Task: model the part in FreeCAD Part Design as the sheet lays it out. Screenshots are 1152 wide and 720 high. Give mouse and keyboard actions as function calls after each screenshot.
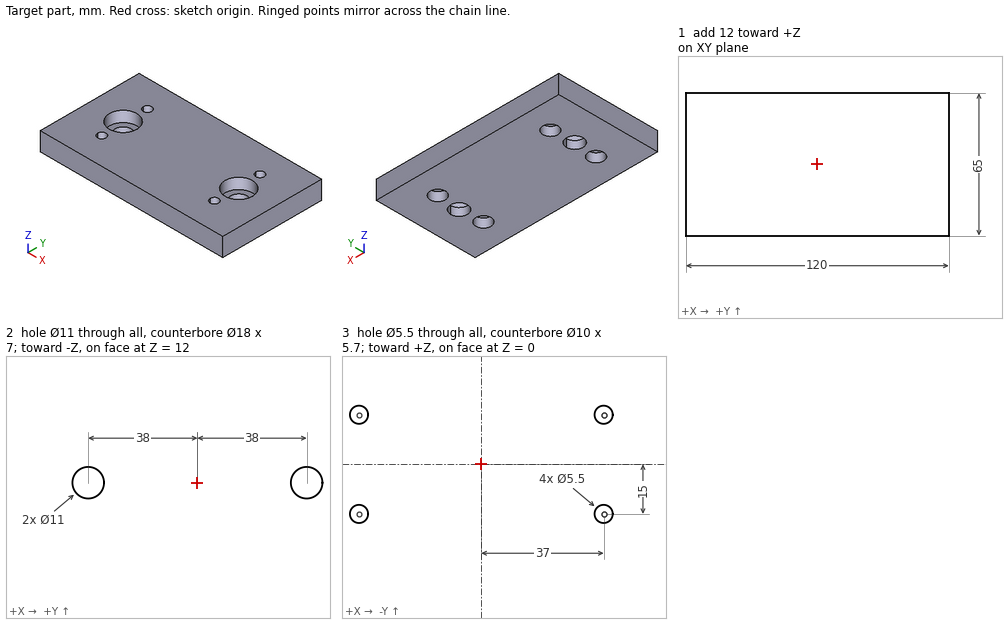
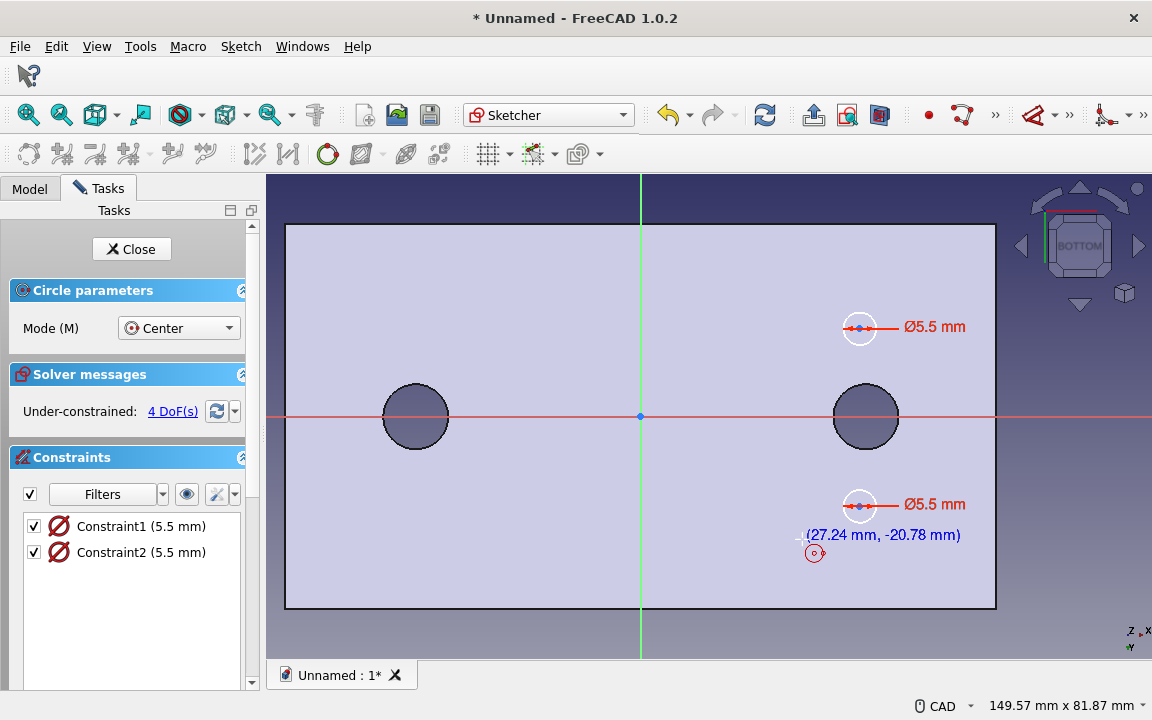
scroll(422, 328, up, 2)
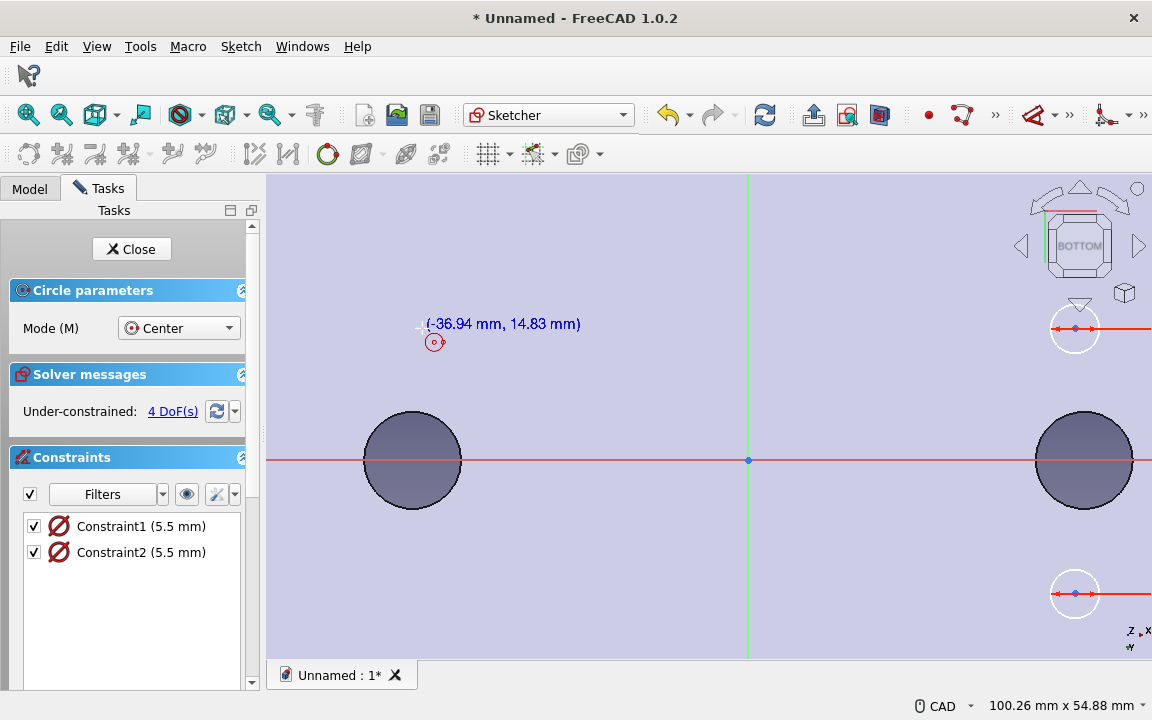
click(421, 328)
move(439, 311)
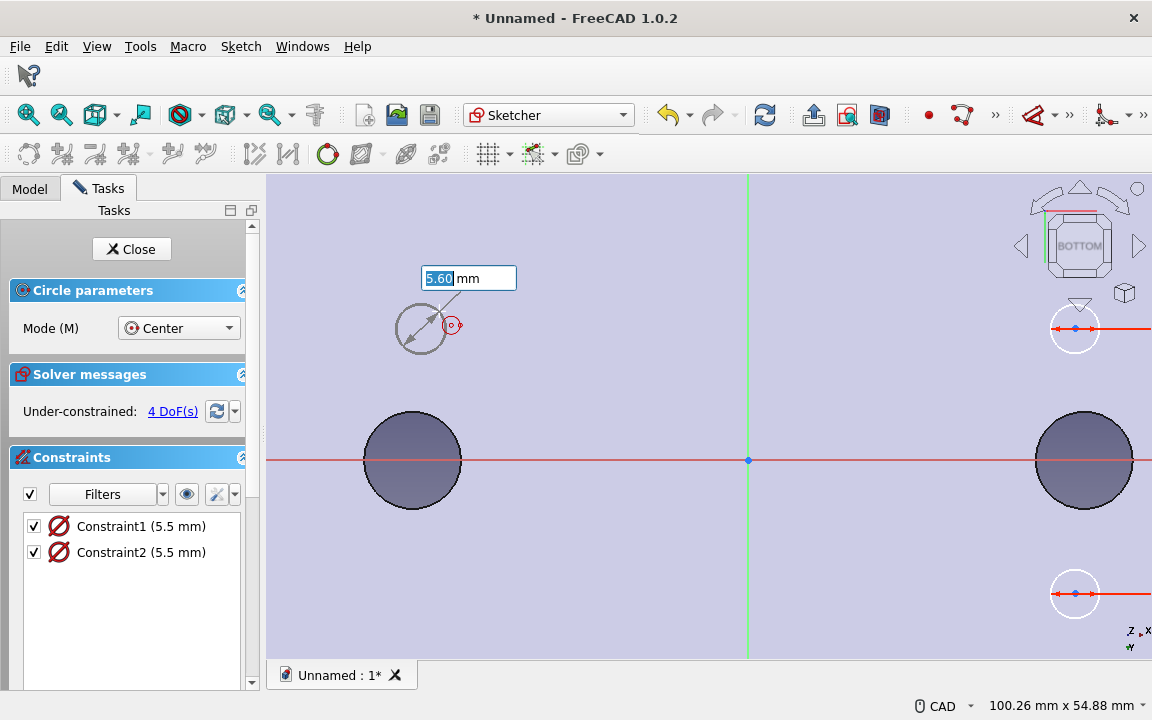
text(5.5)
key(Return)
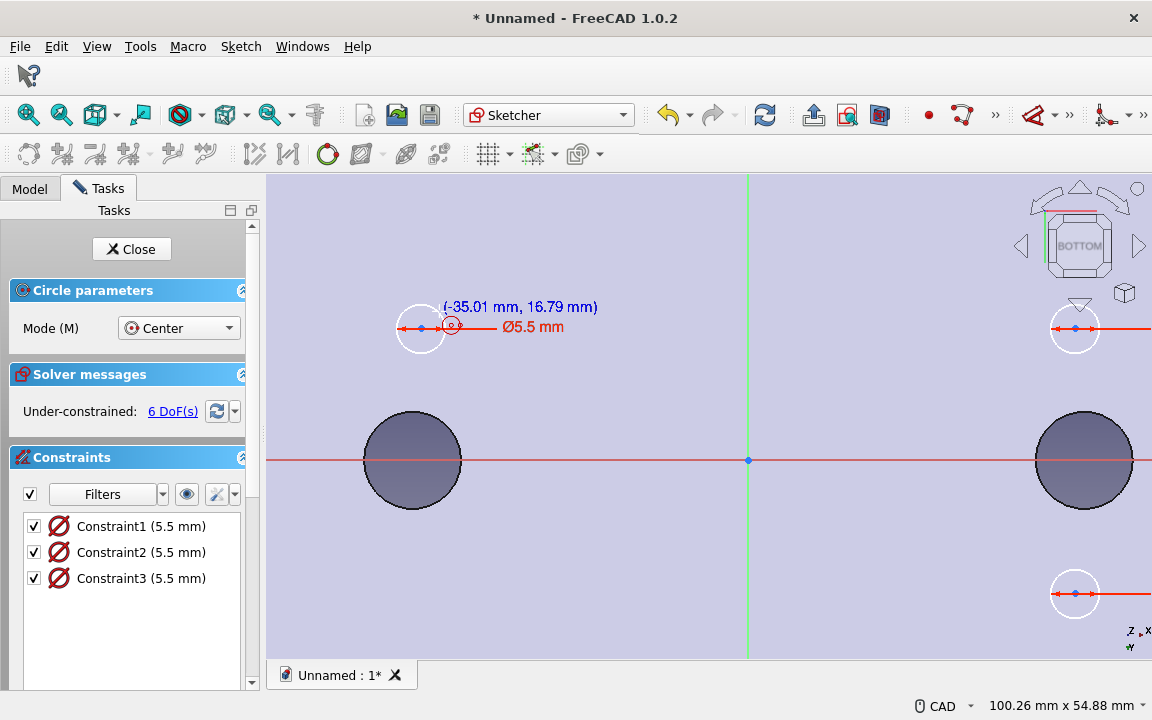
click(421, 593)
move(439, 576)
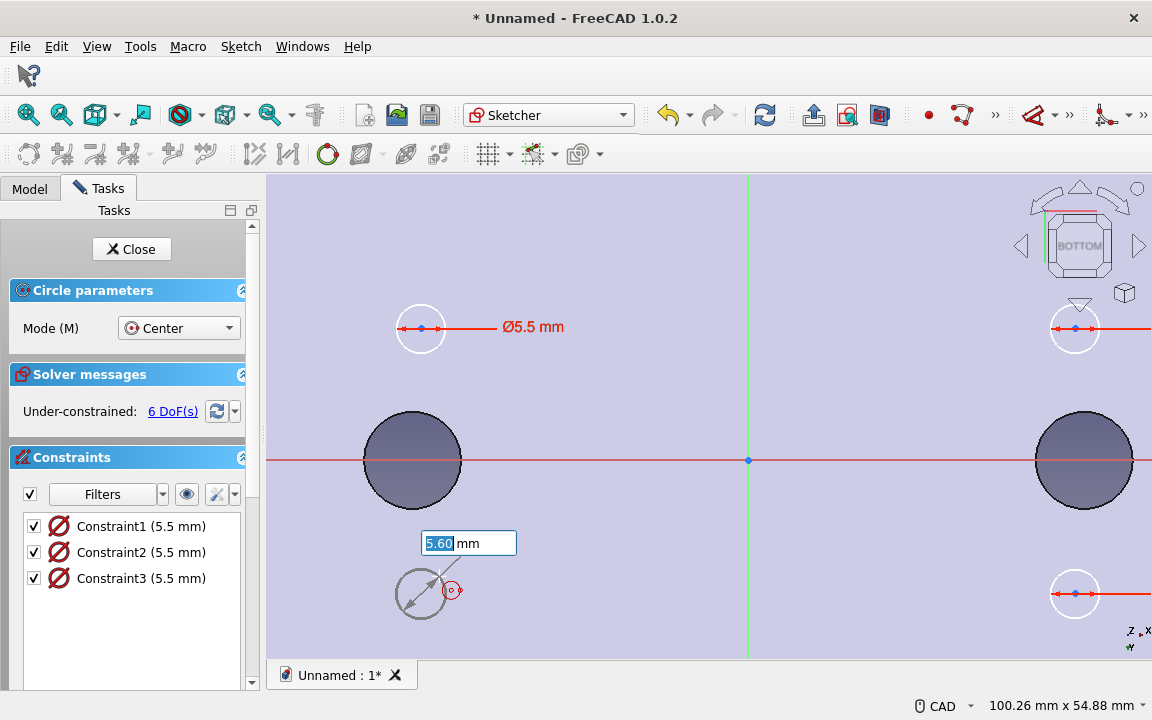
text(5.5)
key(Return)
key(Escape)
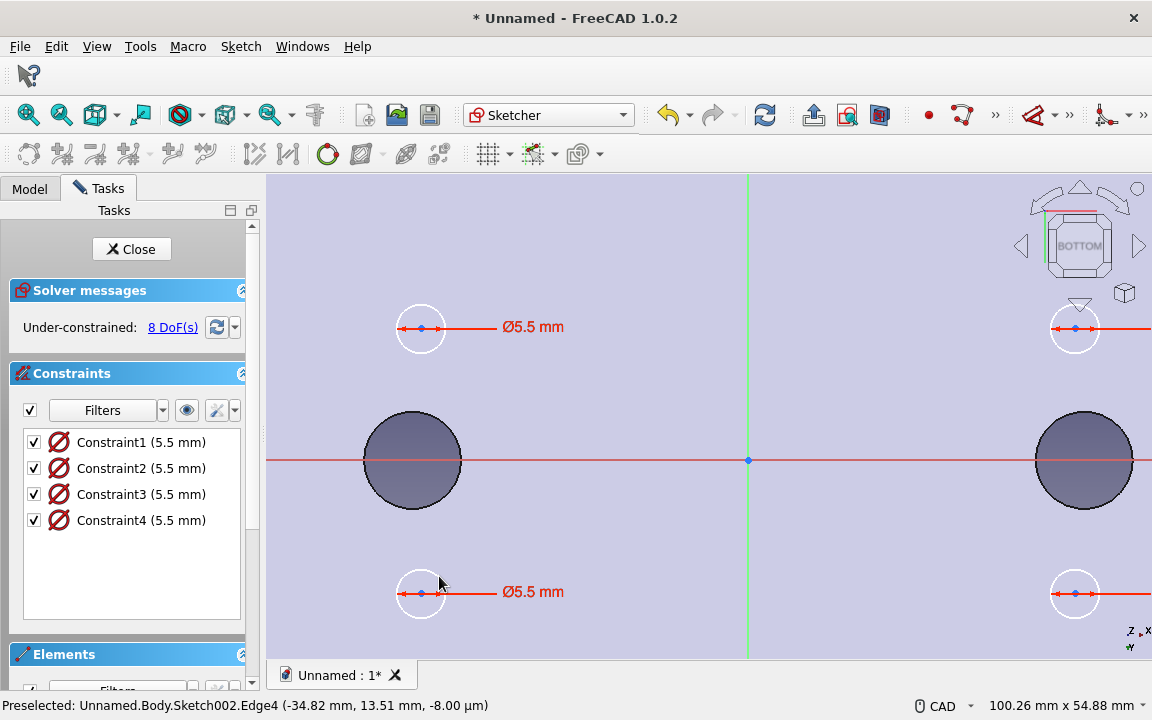
scroll(421, 327, down, 2)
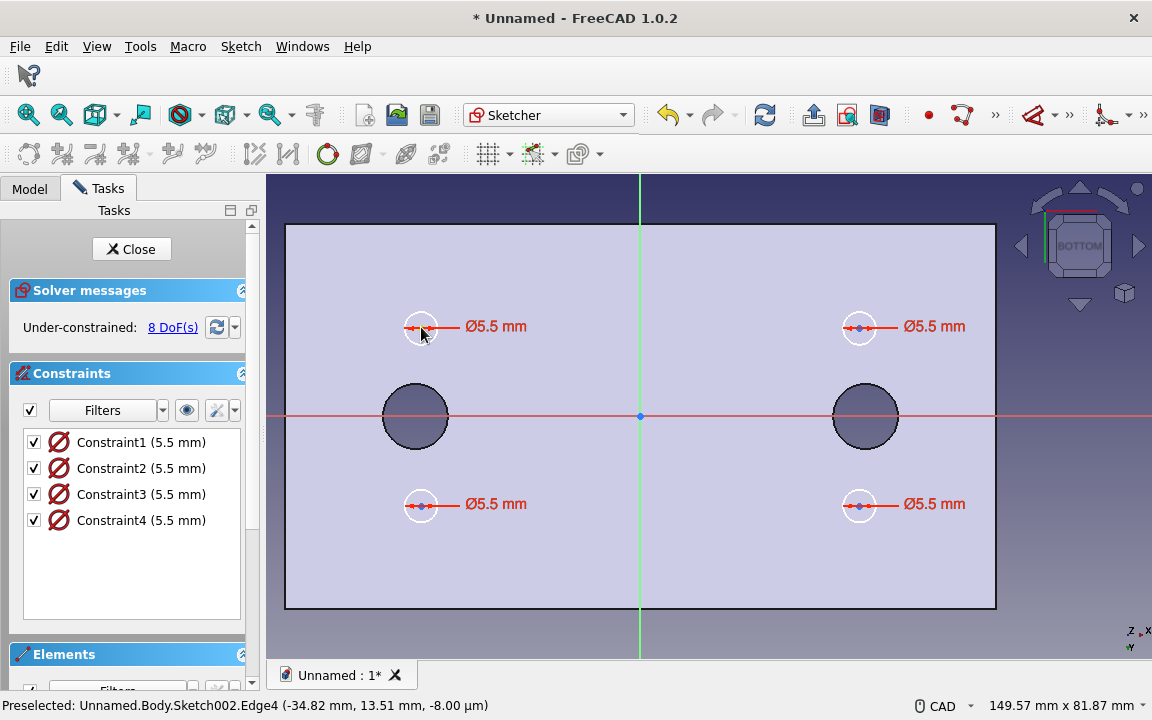
click(860, 506)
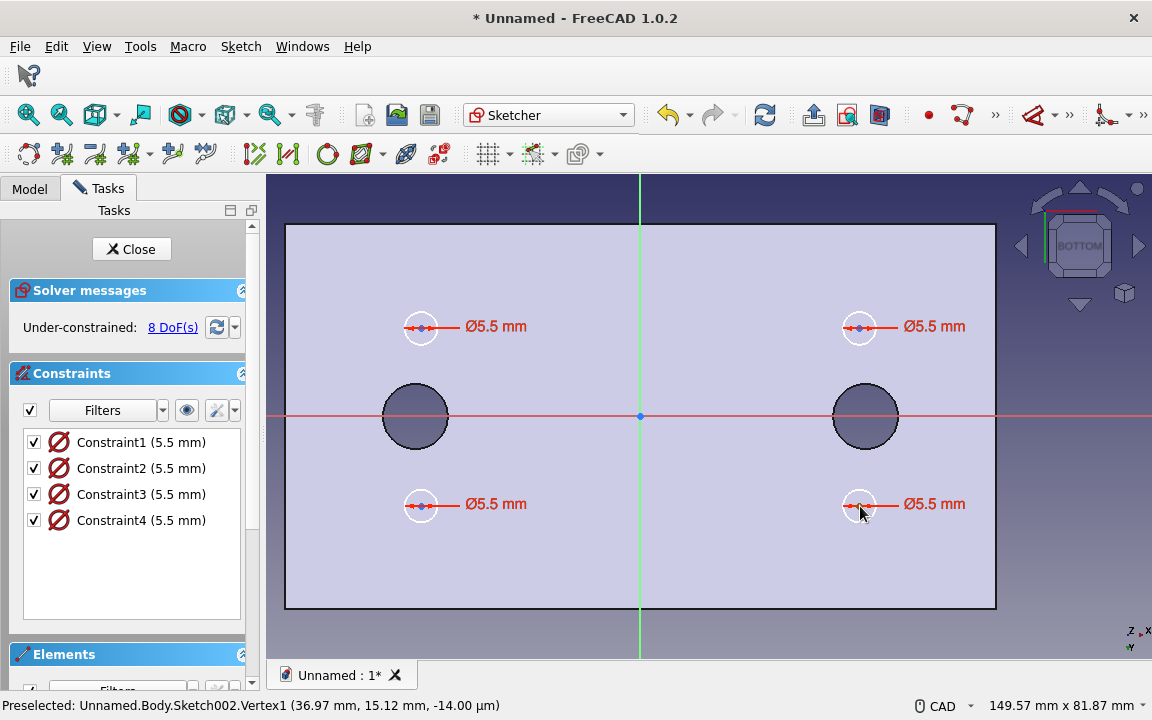
click(860, 328)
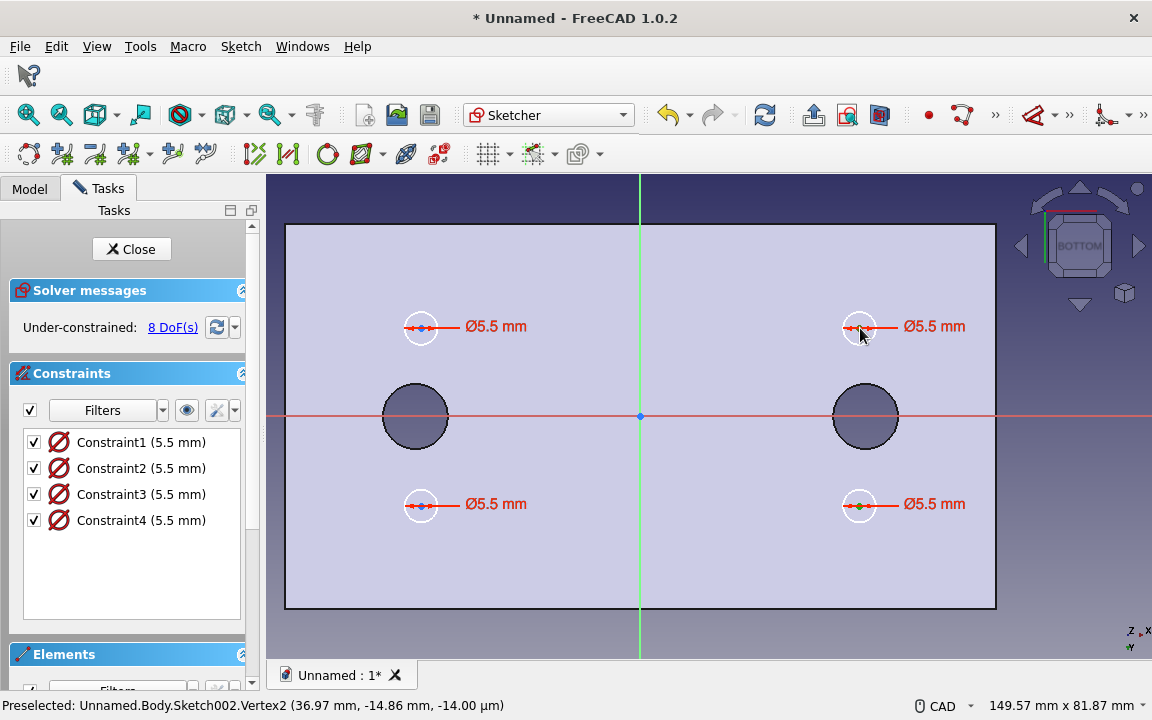
click(344, 416)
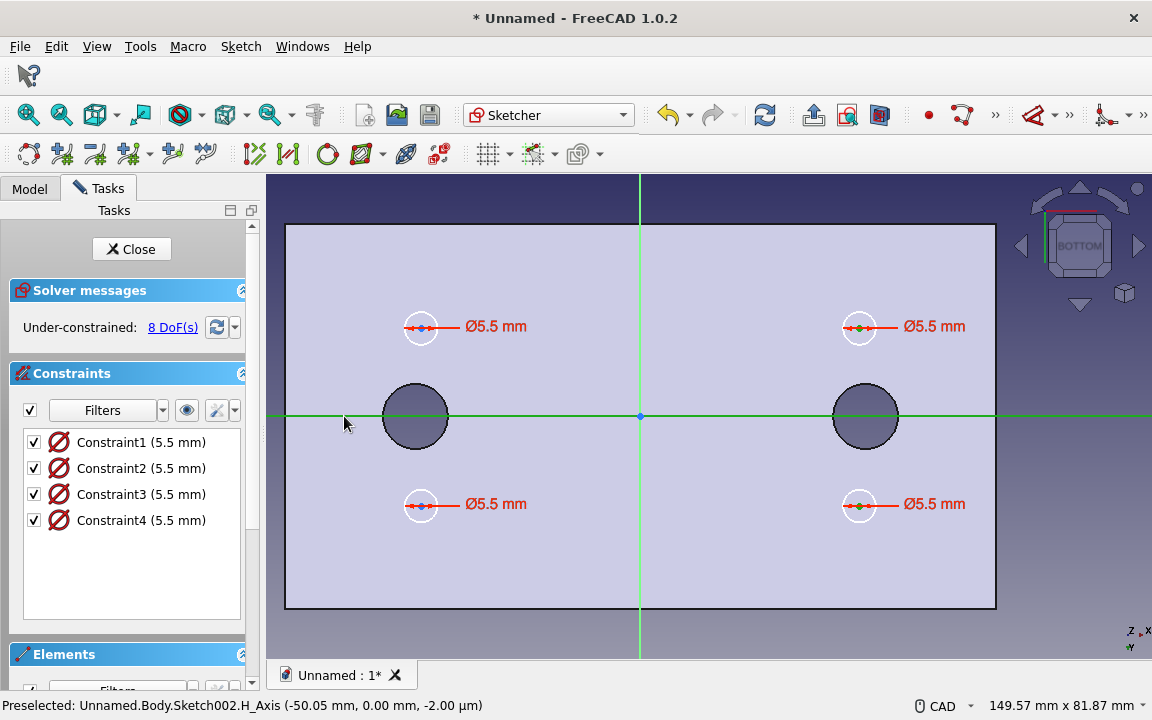
key(s)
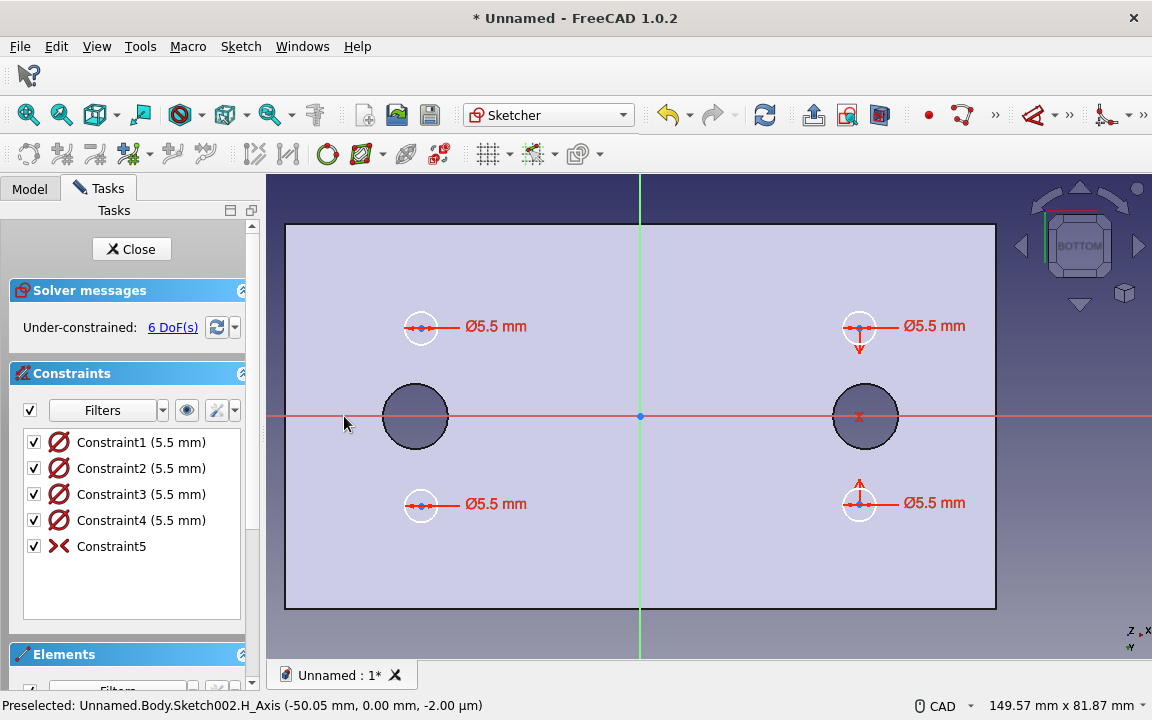
click(860, 328)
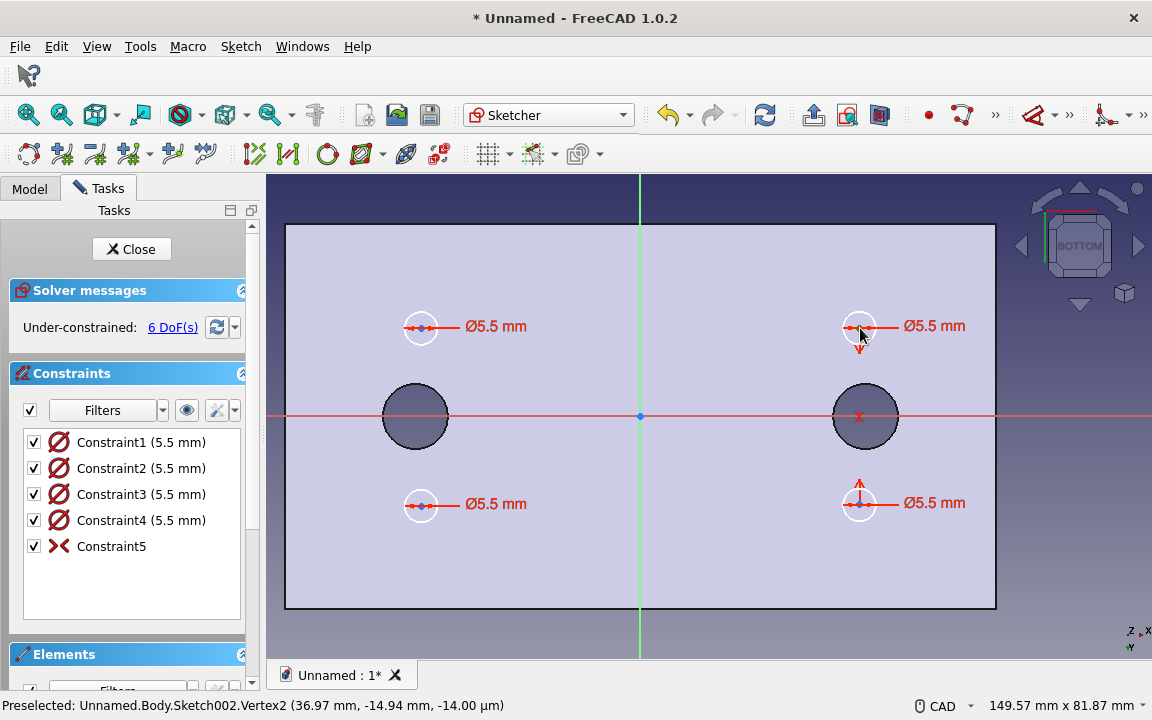
click(421, 328)